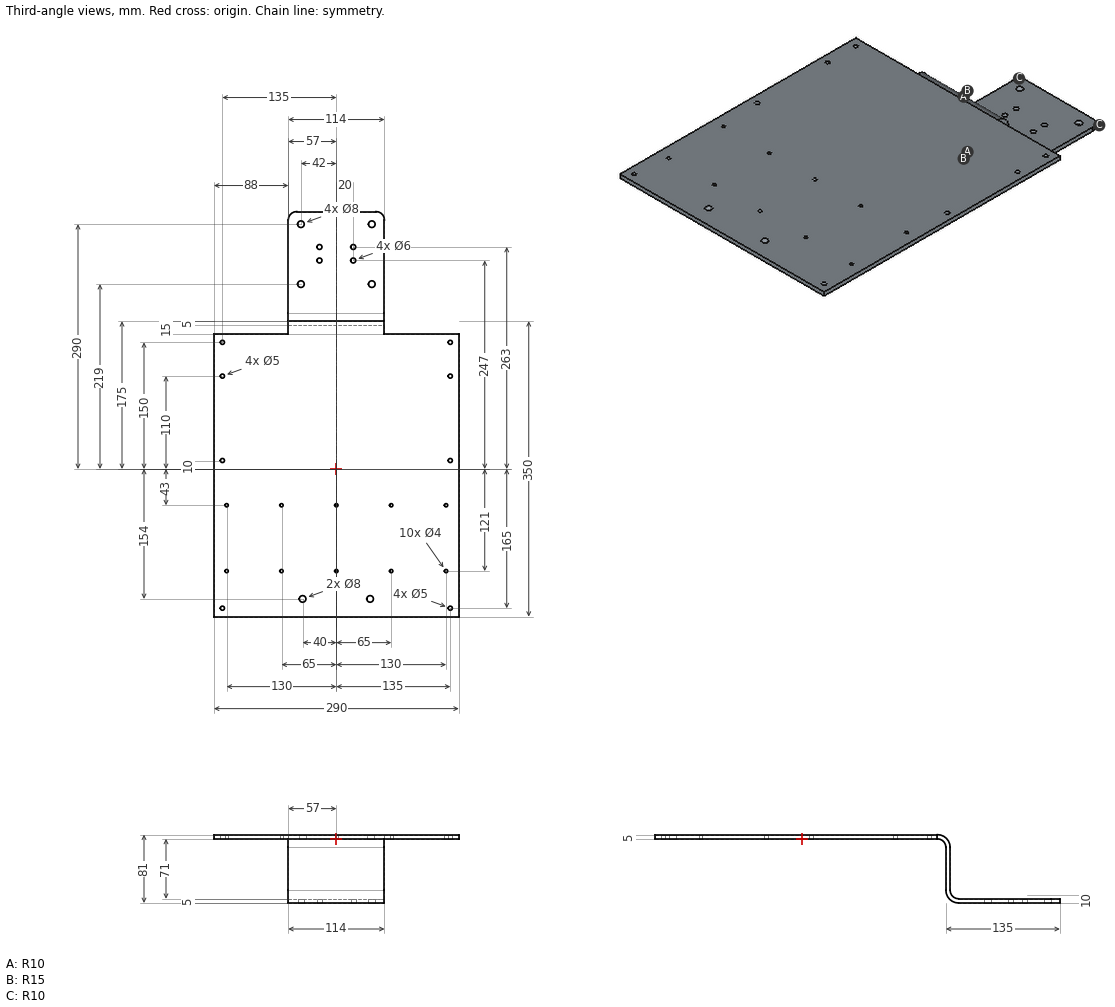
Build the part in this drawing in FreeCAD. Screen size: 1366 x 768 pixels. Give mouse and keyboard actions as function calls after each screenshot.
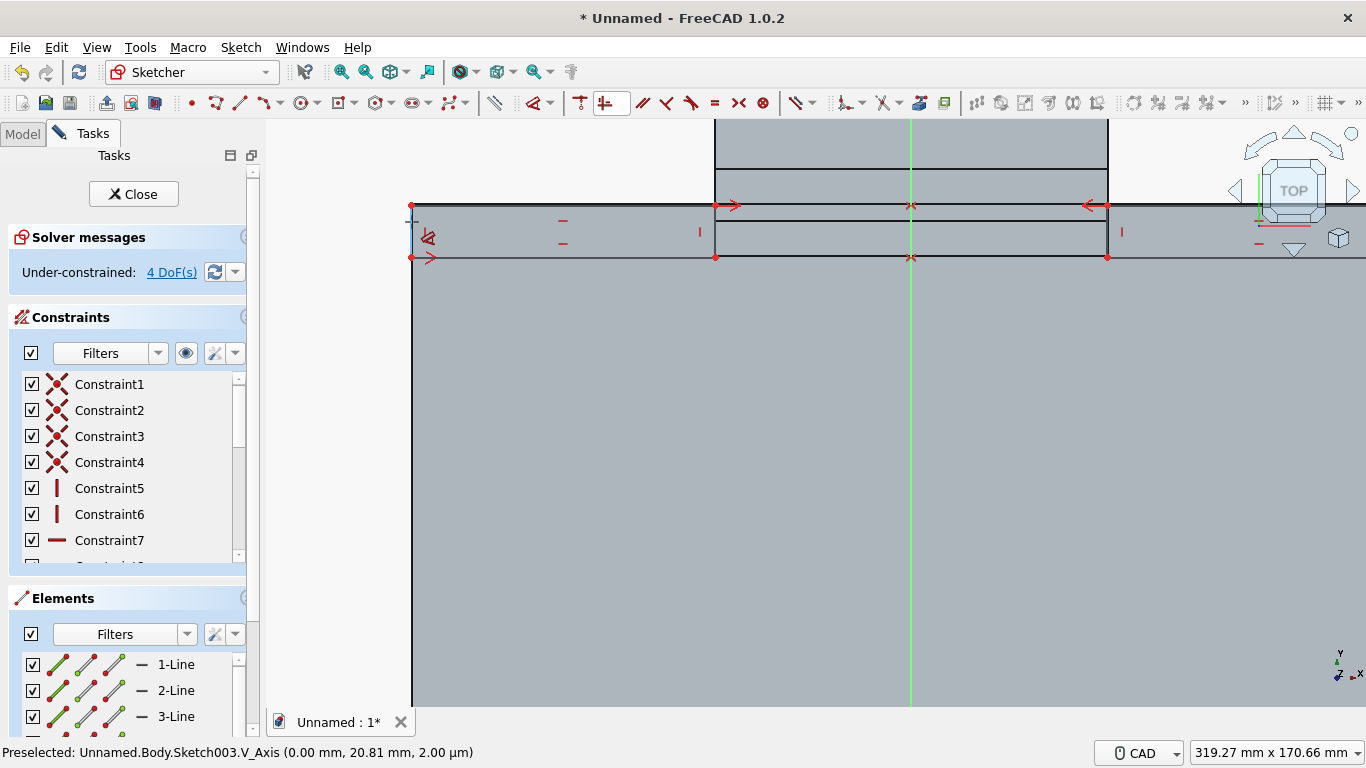
click(411, 221)
click(377, 232)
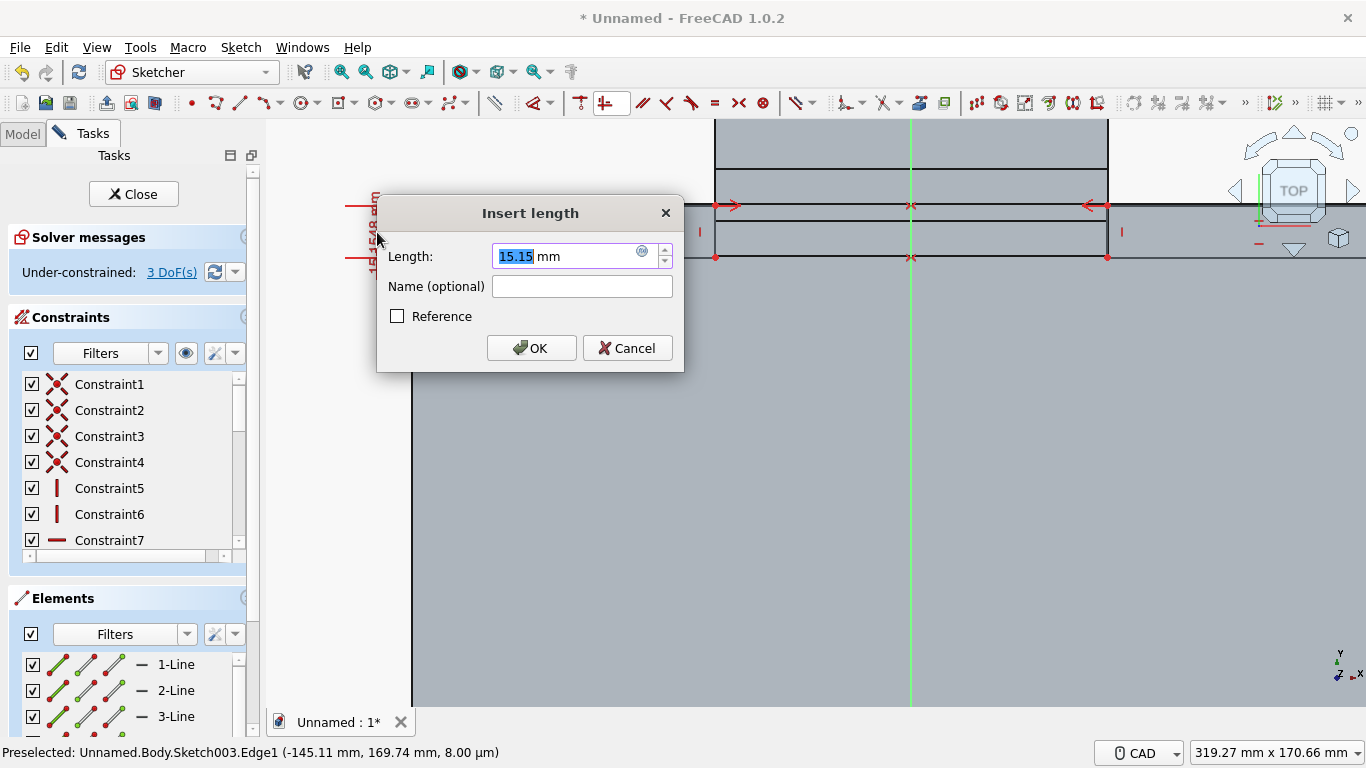
text(15)
key(Return)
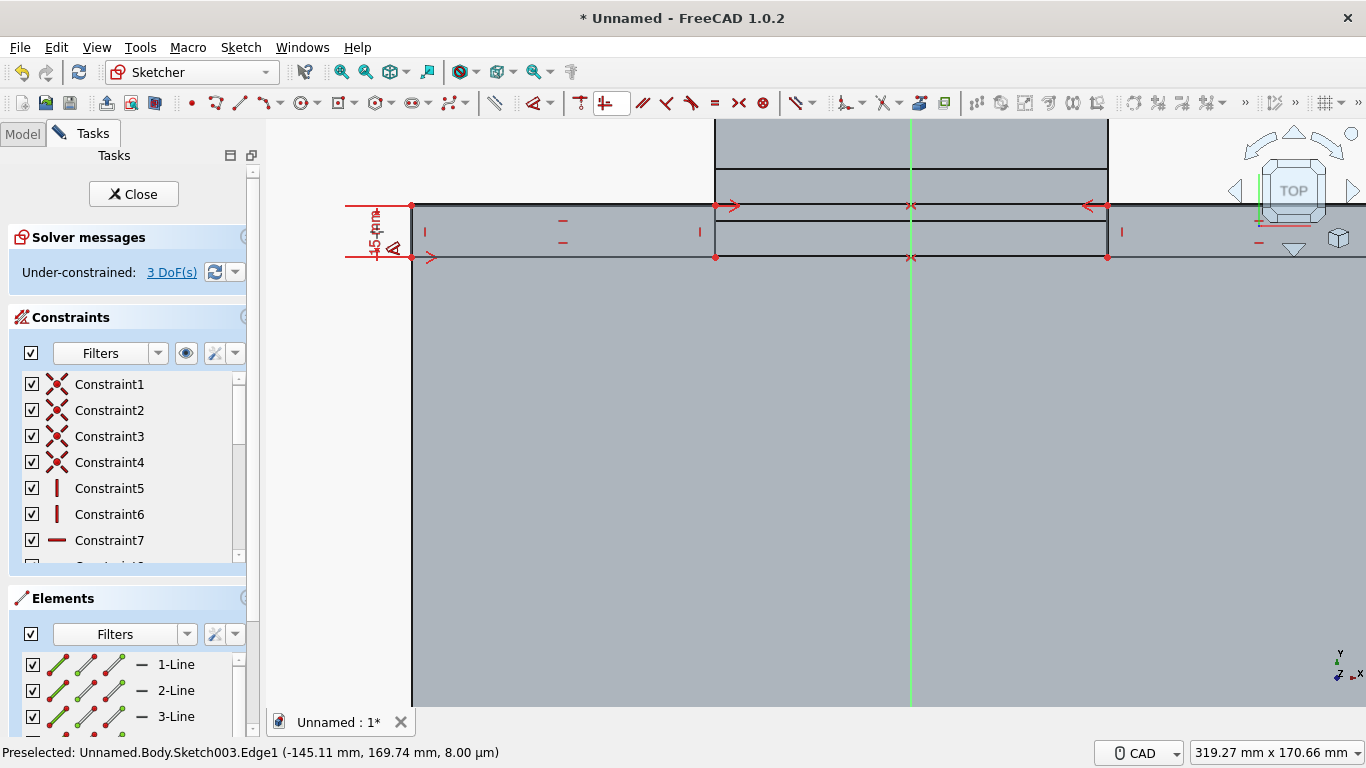
click(502, 257)
click(563, 223)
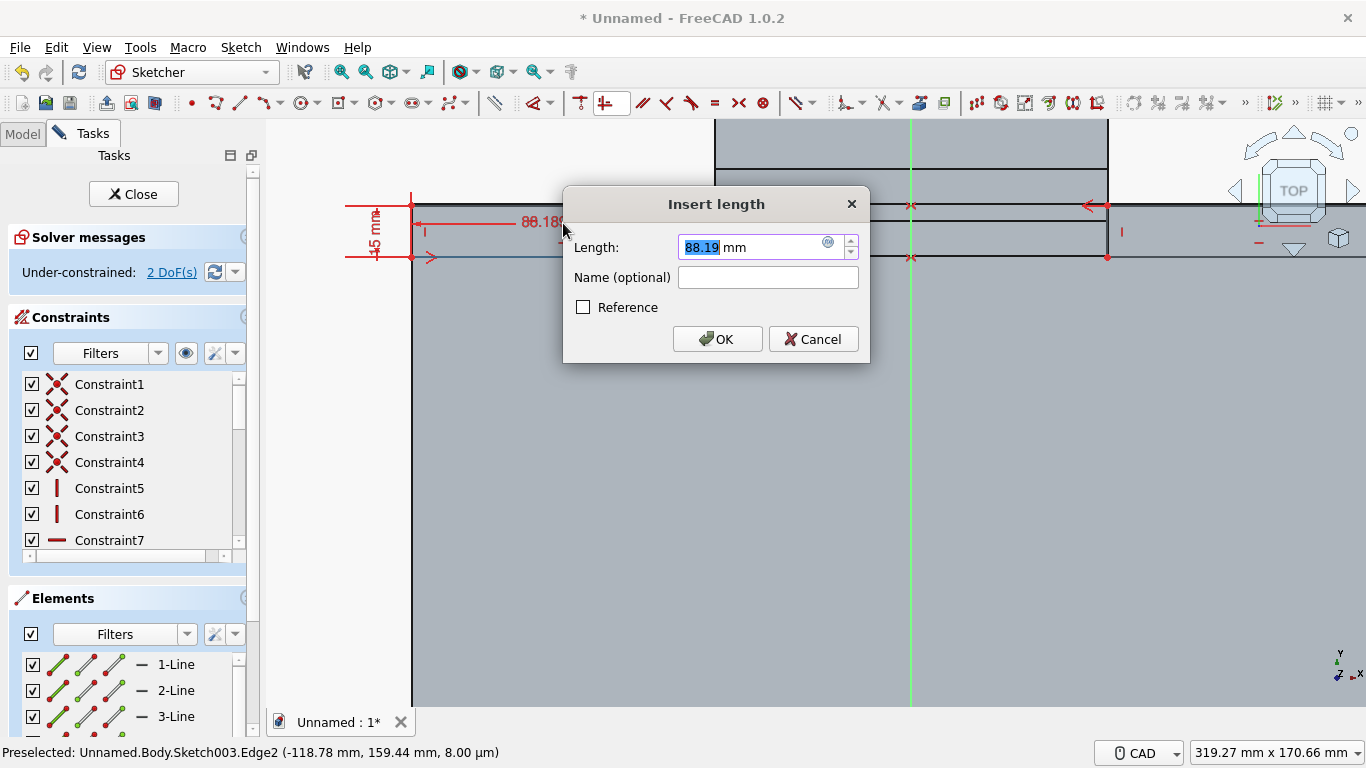
text(88)
key(Return)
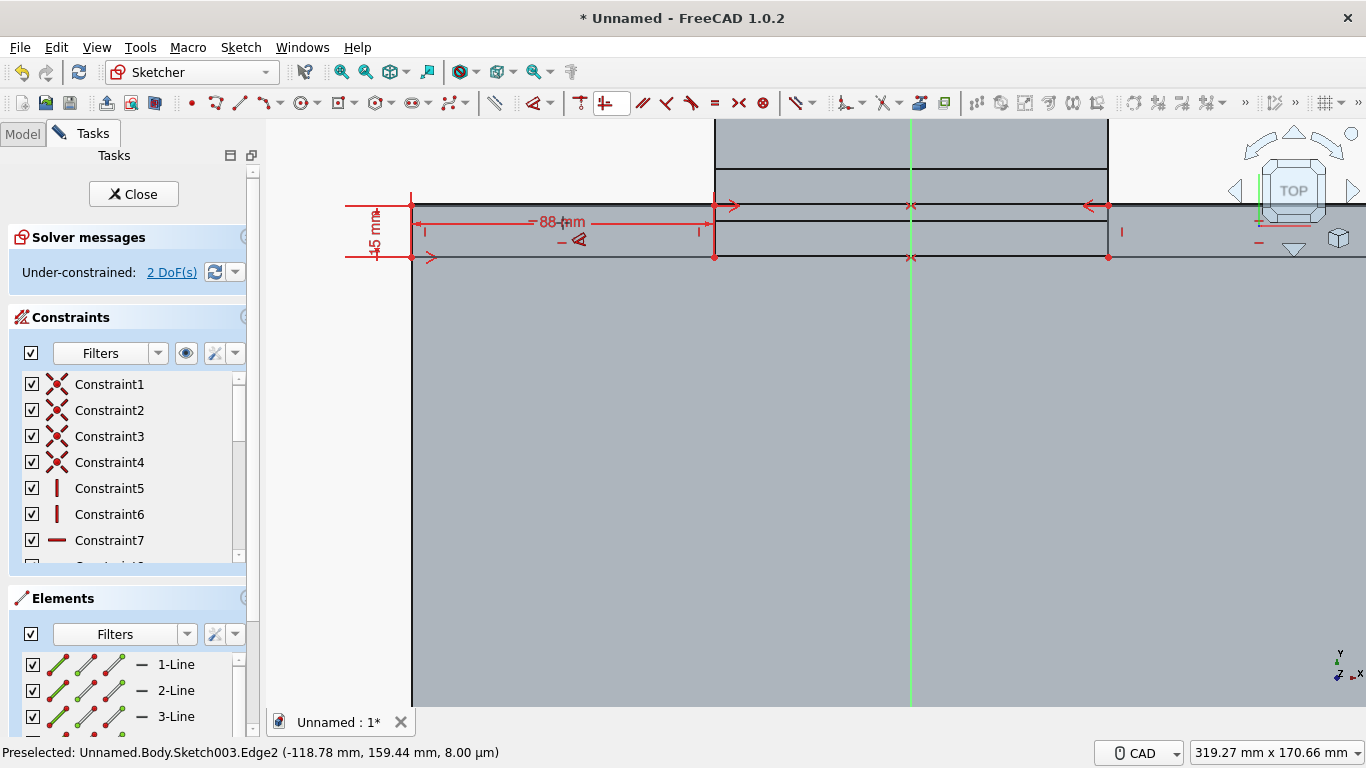
click(714, 257)
click(813, 223)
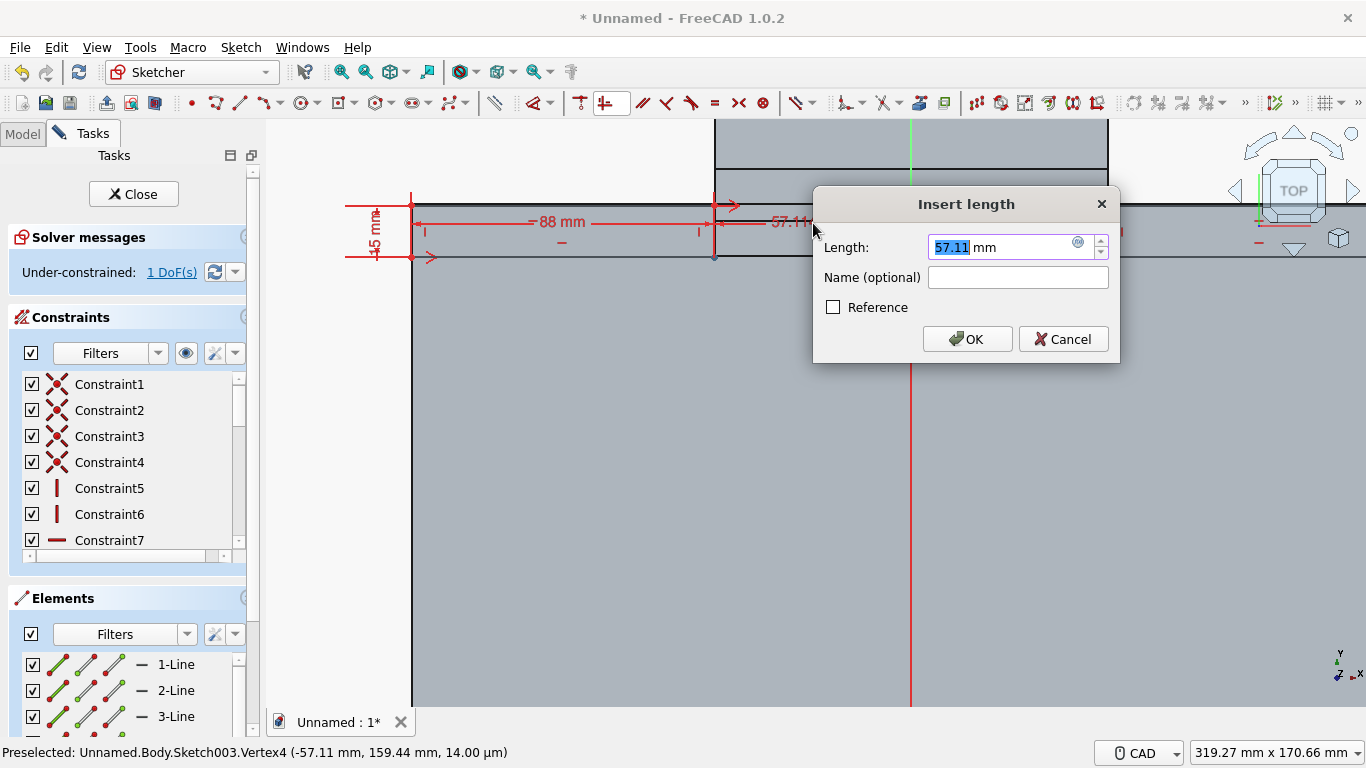
text(57)
key(Return)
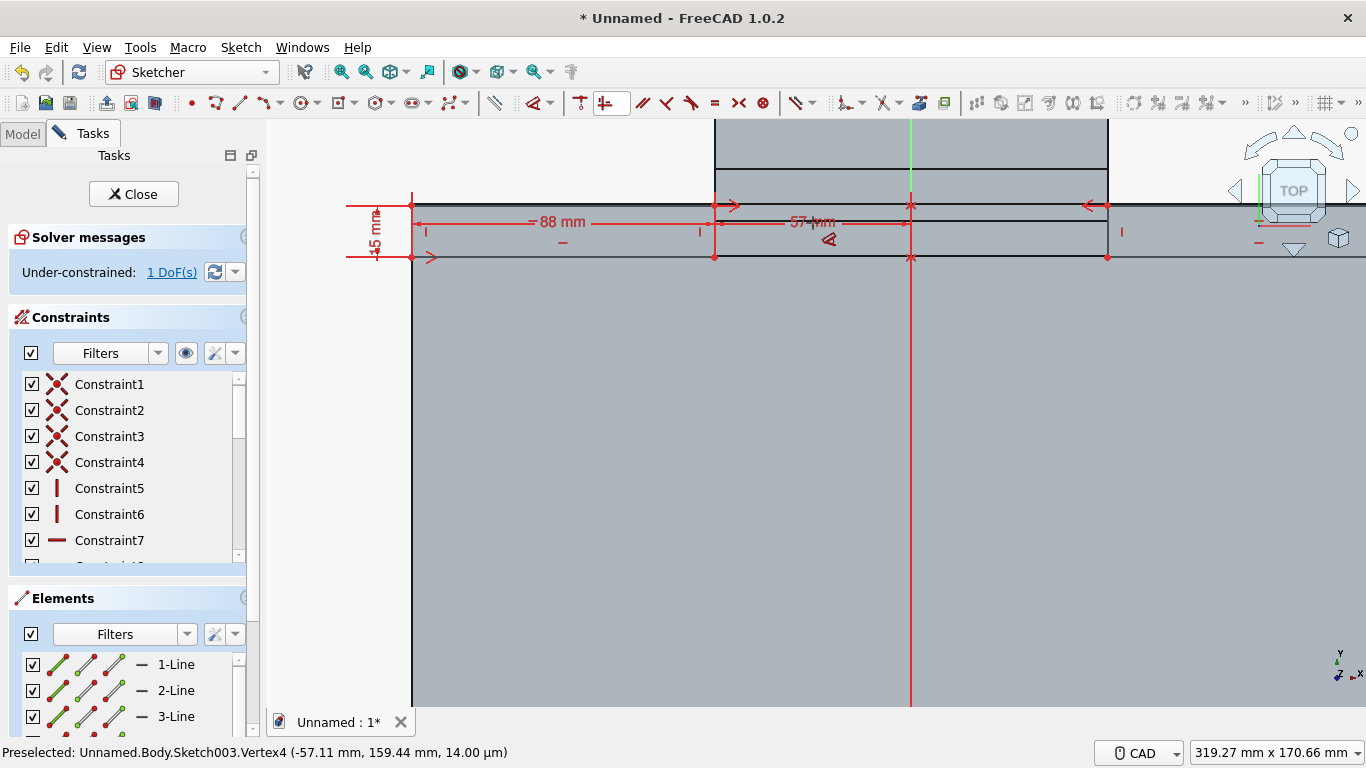
click(412, 206)
click(378, 442)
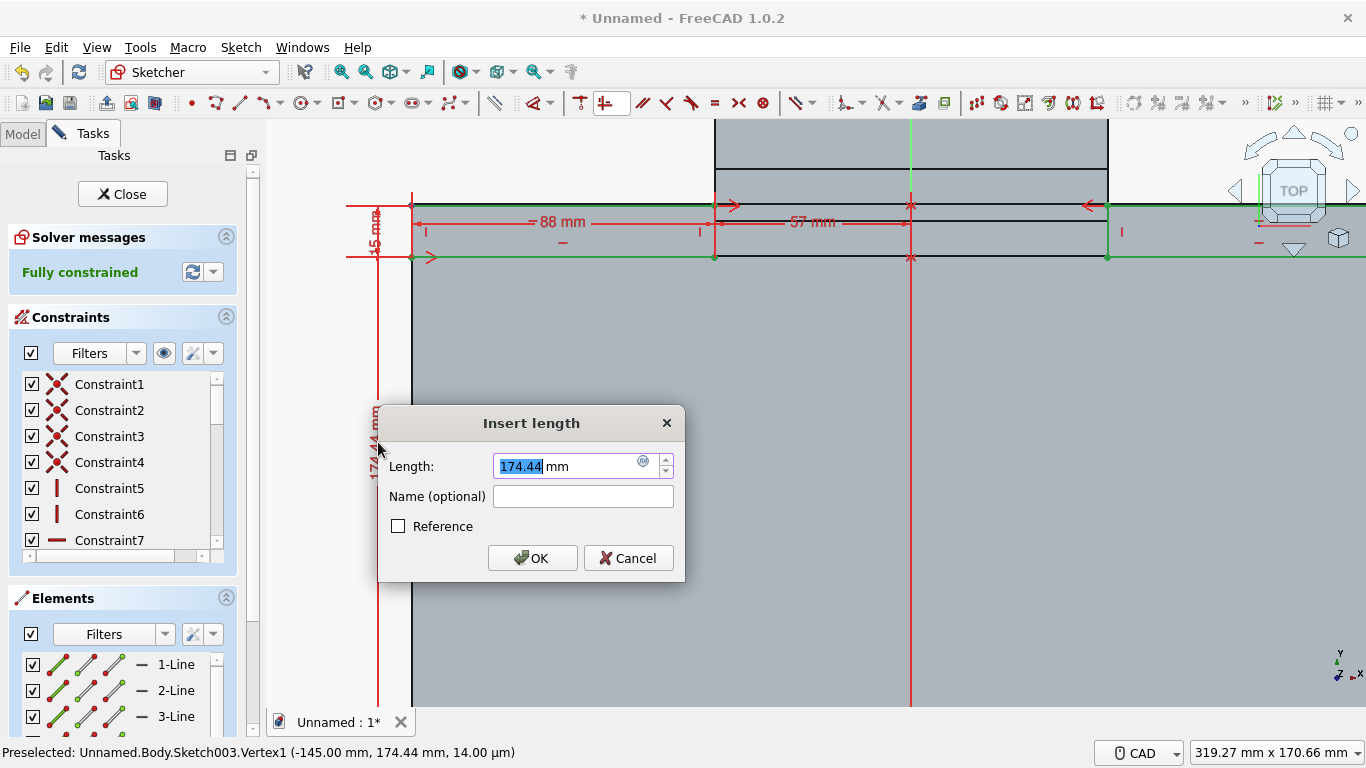
text(175)
key(Return)
key(Escape)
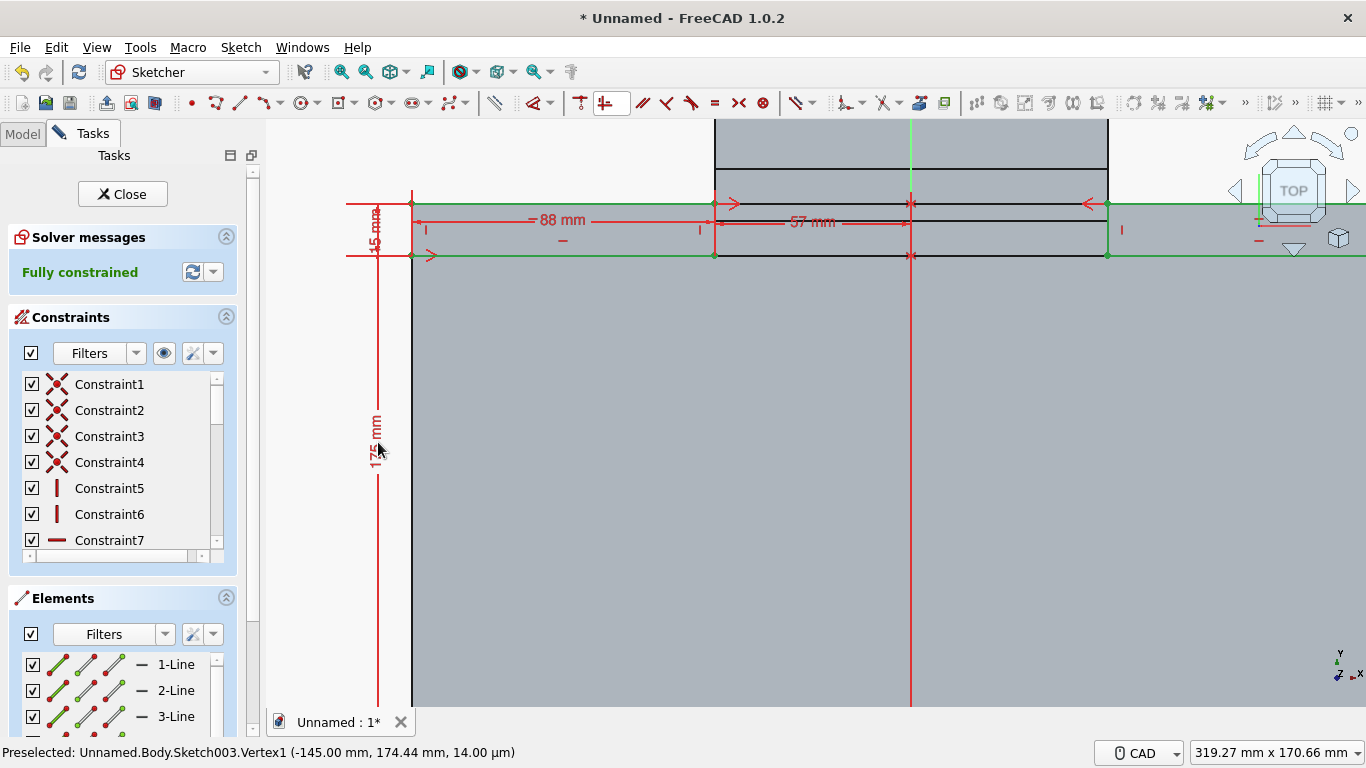
click(123, 194)